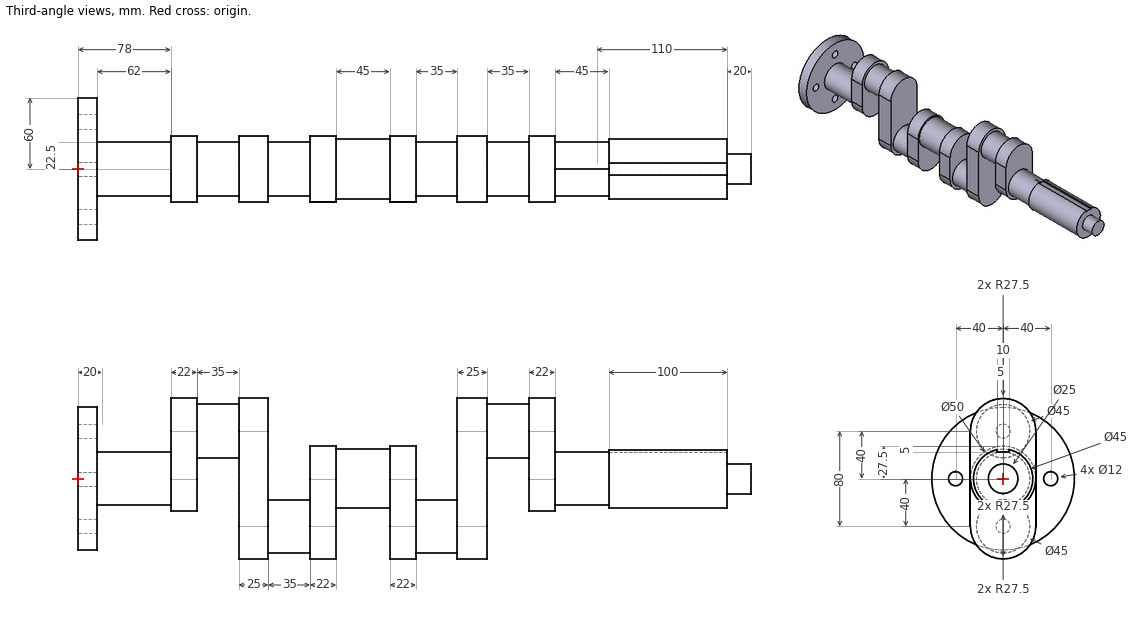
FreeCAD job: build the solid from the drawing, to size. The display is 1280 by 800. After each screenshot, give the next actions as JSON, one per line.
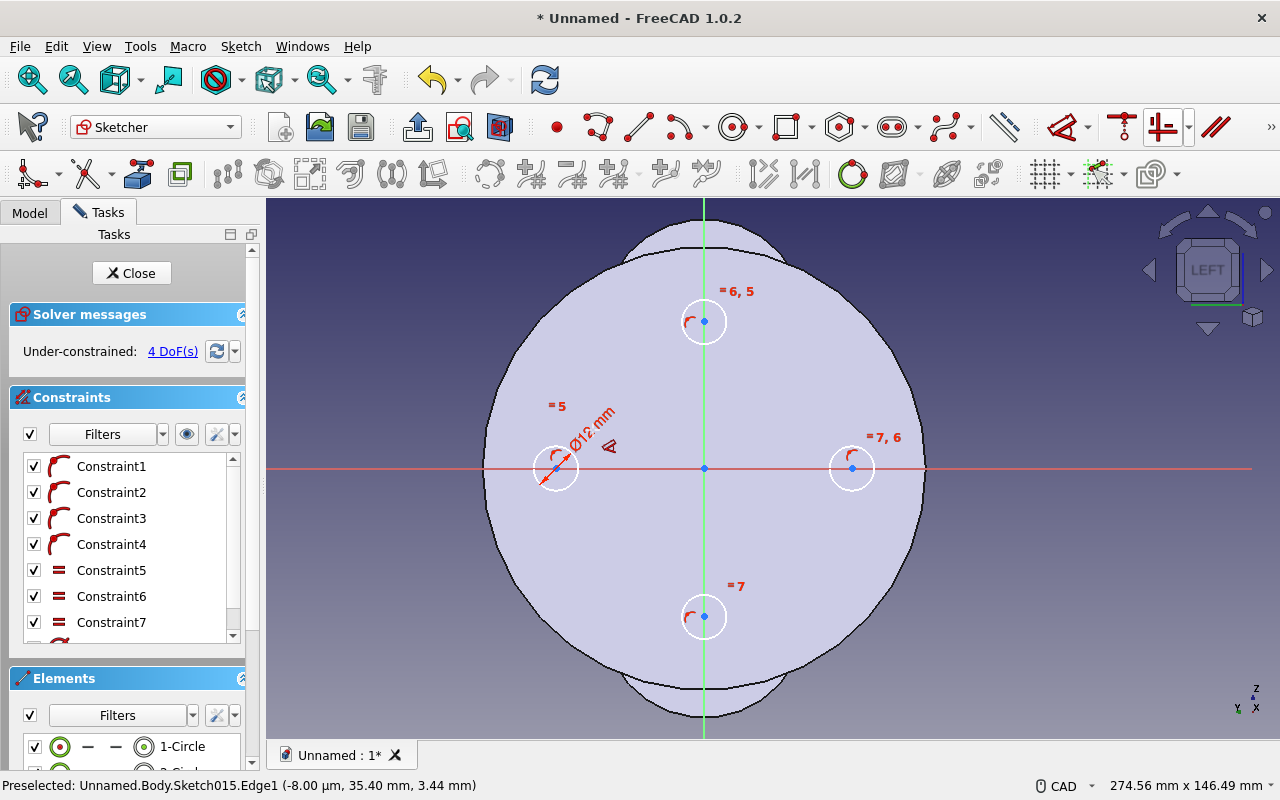
{"action": "left_click", "coordinate": [556, 468]}
{"action": "left_click", "coordinate": [630, 502]}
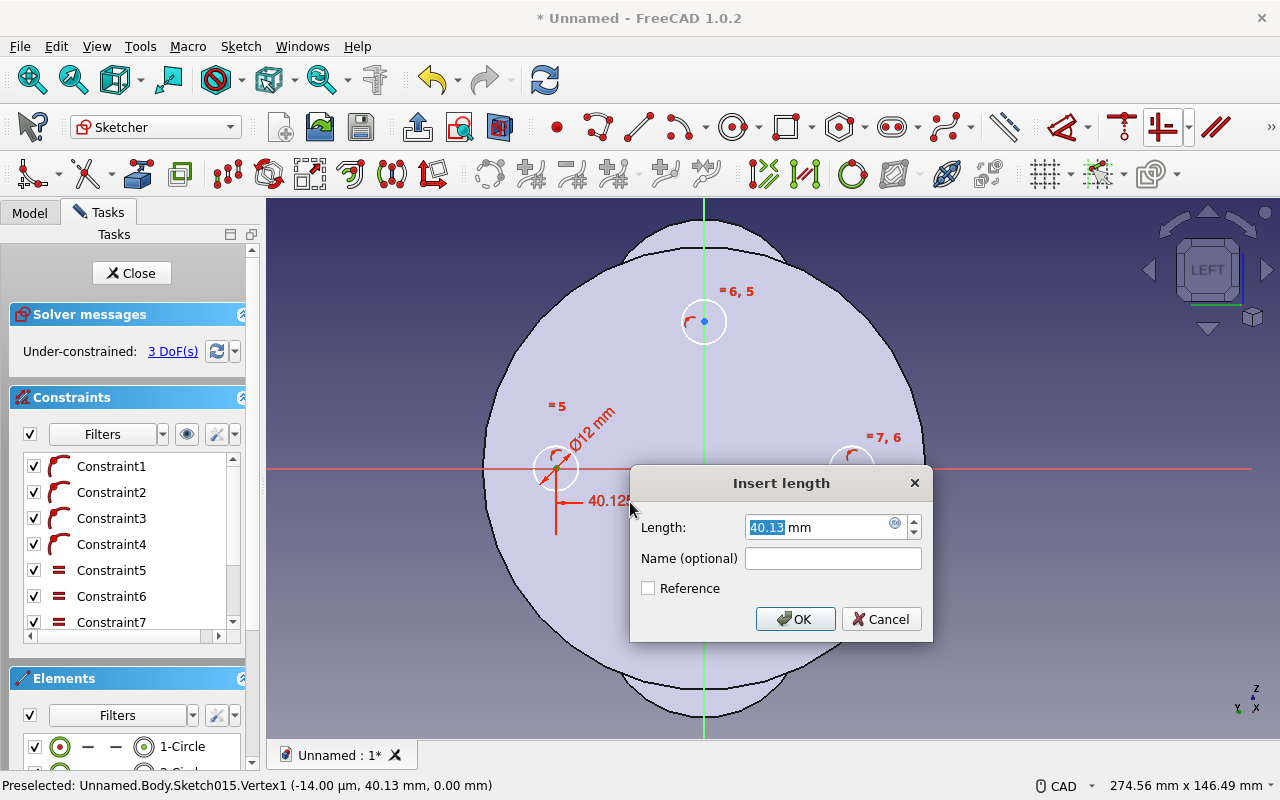
{"action": "type", "text": "40"}
{"action": "key", "text": "Return"}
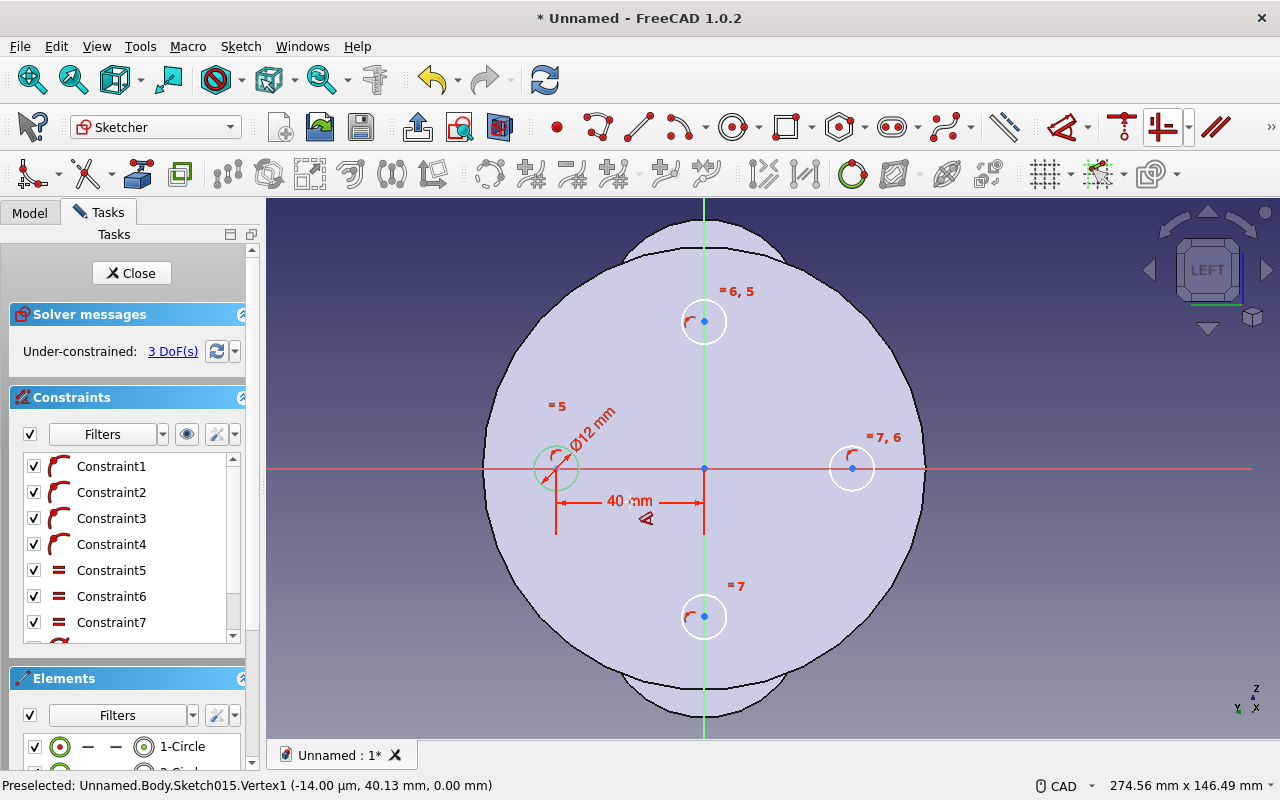
{"action": "left_click", "coordinate": [704, 322]}
{"action": "left_click", "coordinate": [738, 395]}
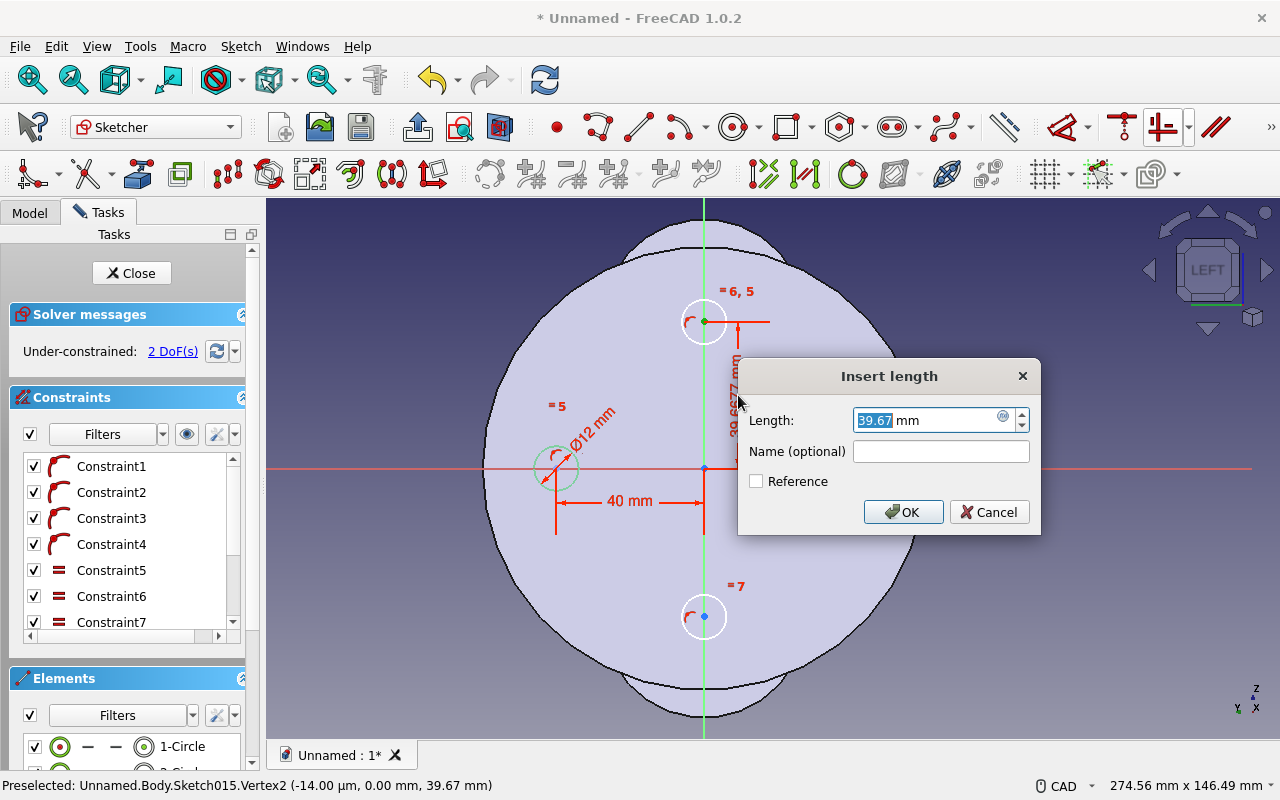
{"action": "type", "text": "40"}
{"action": "key", "text": "Return"}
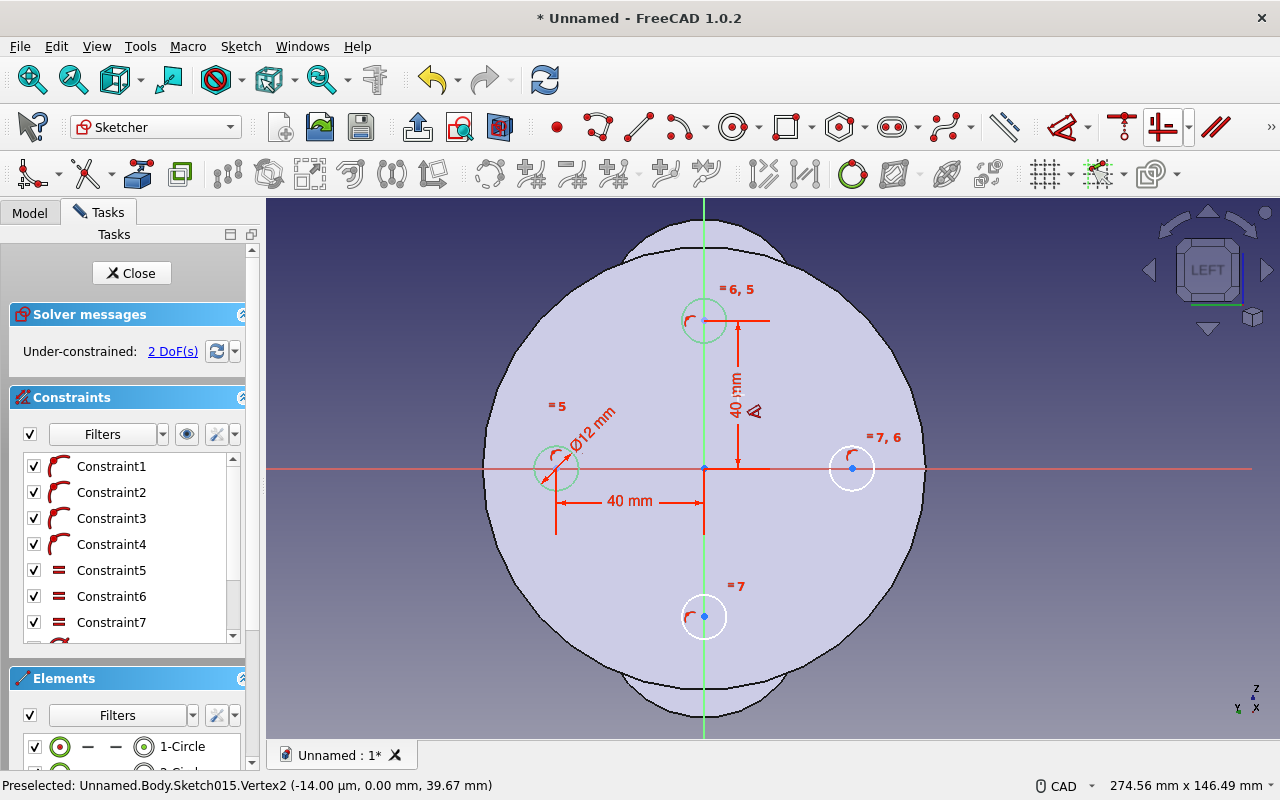
{"action": "left_click", "coordinate": [852, 468]}
{"action": "left_click", "coordinate": [778, 502]}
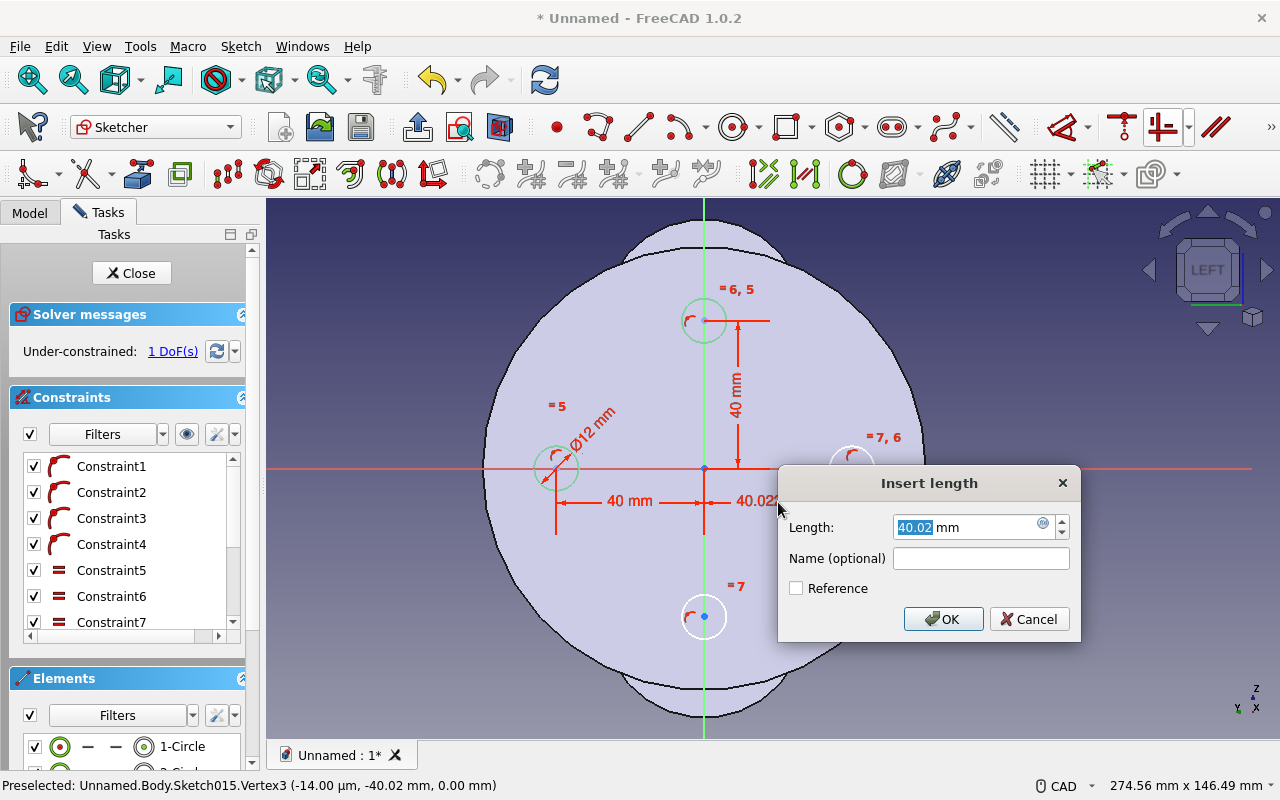
{"action": "type", "text": "40"}
{"action": "key", "text": "Return"}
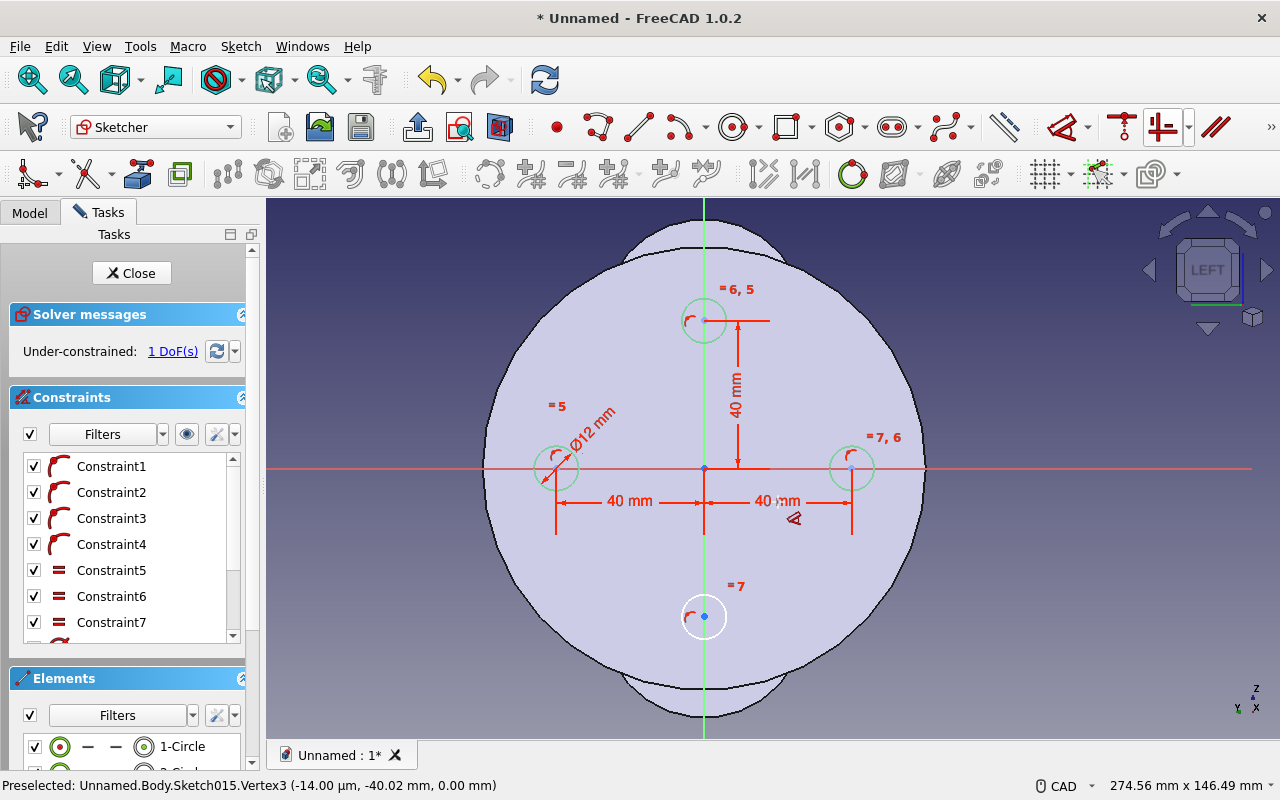
{"action": "left_click", "coordinate": [704, 617]}
{"action": "left_click", "coordinate": [738, 543]}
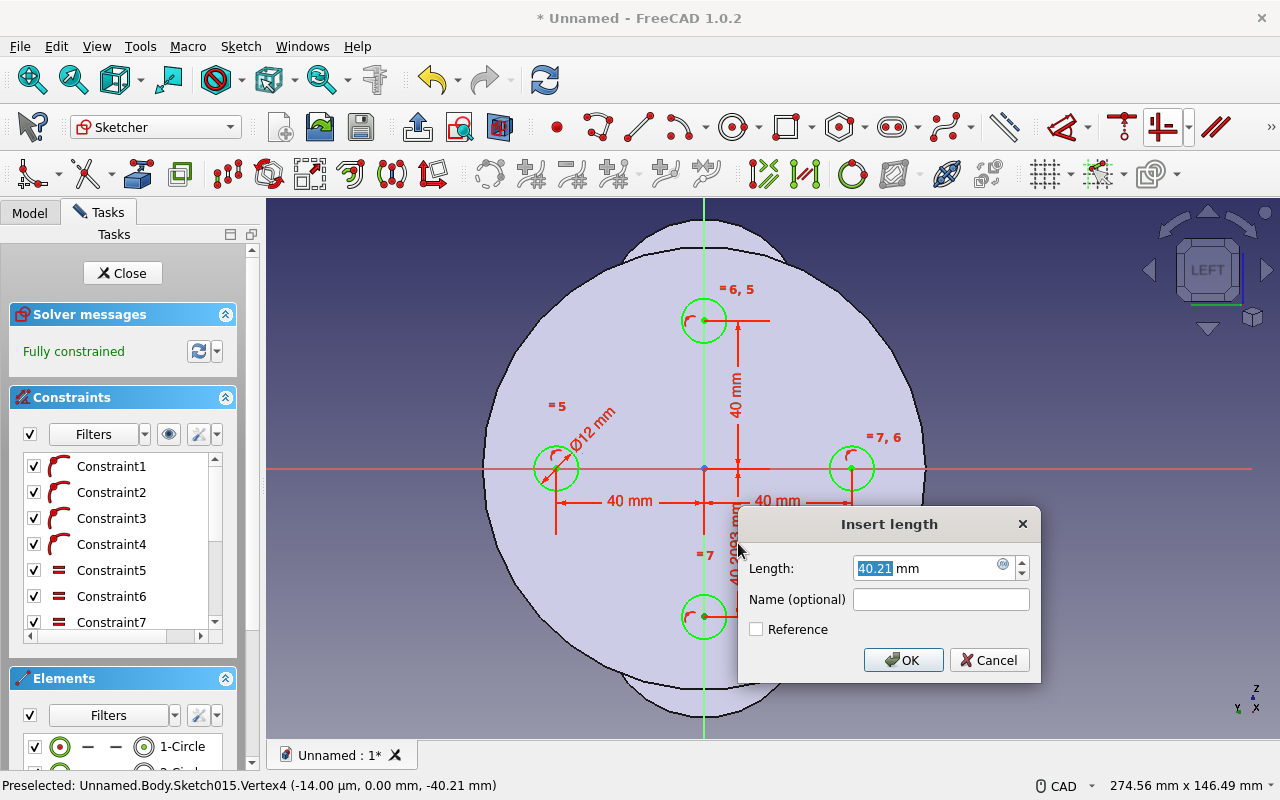
{"action": "type", "text": "40"}
{"action": "key", "text": "Return"}
{"action": "key", "text": "Escape"}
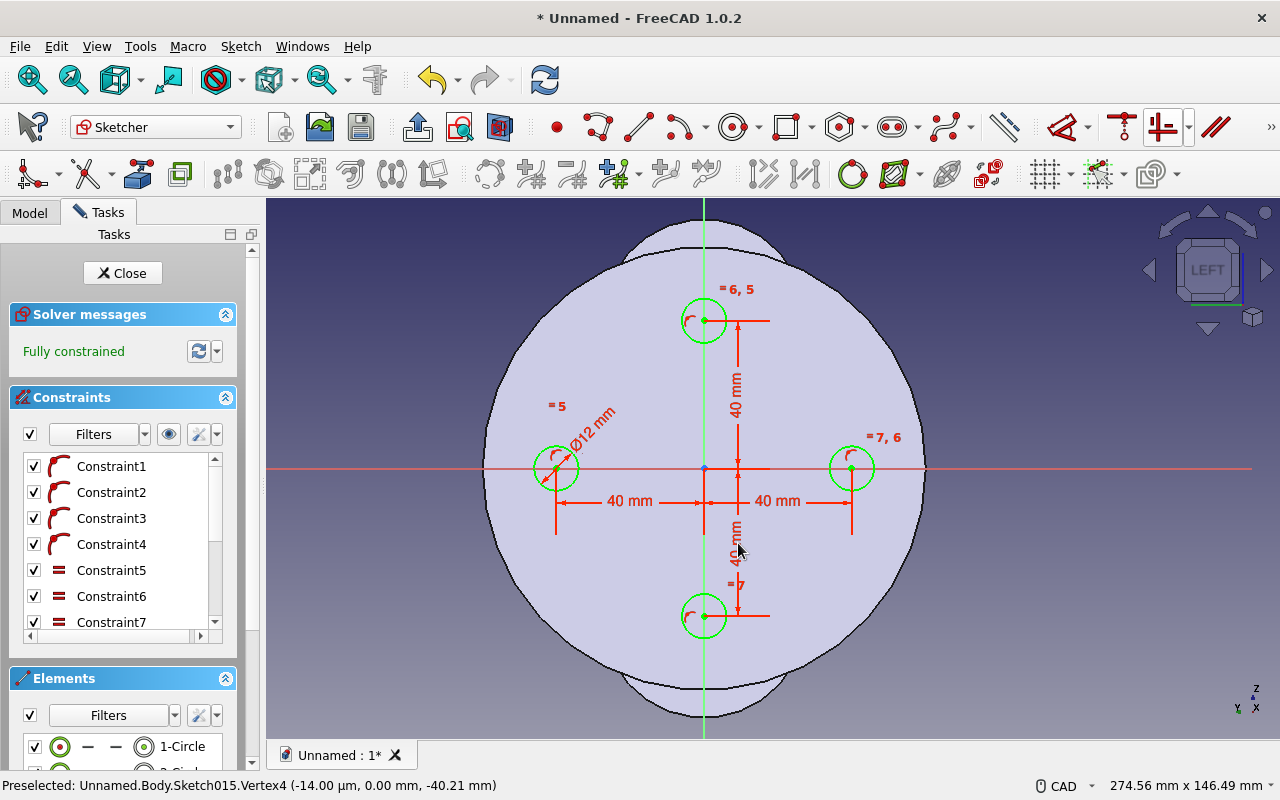
{"action": "left_click", "coordinate": [123, 273]}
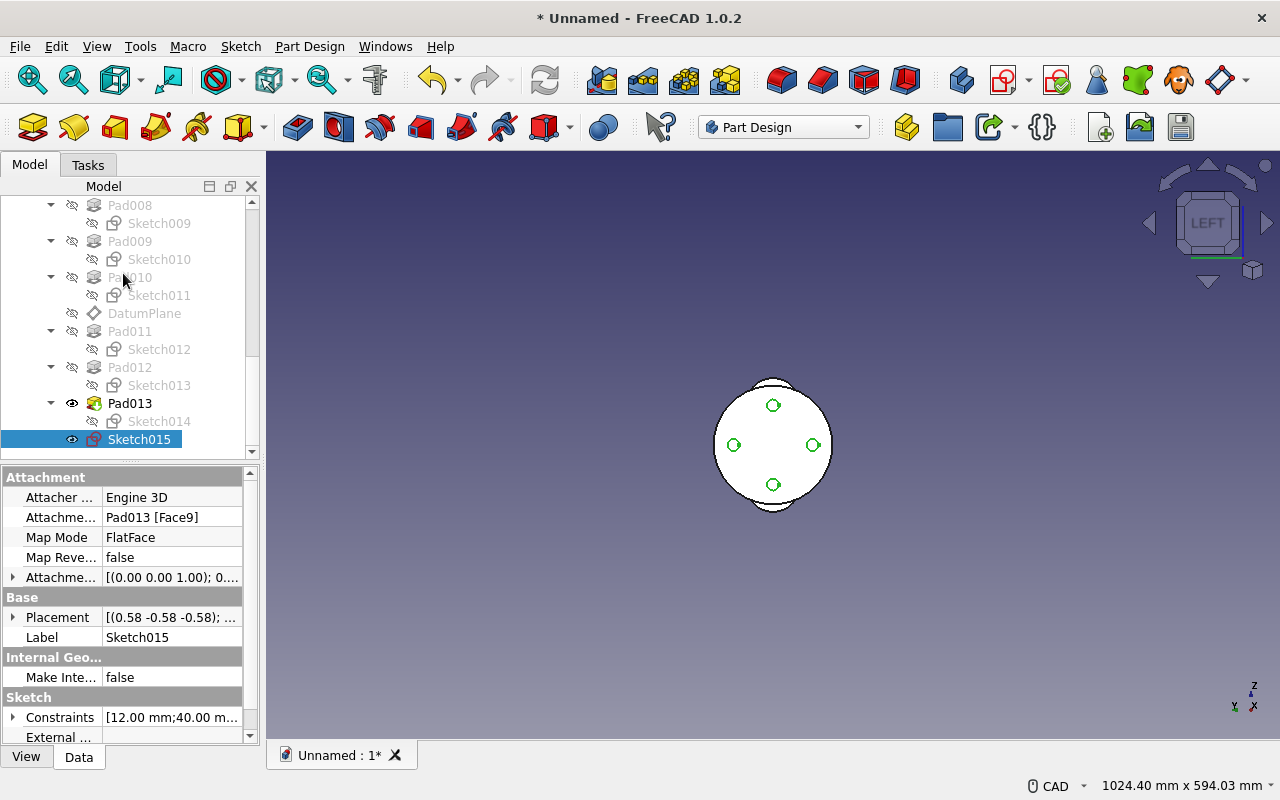
{"action": "left_click", "coordinate": [298, 128]}